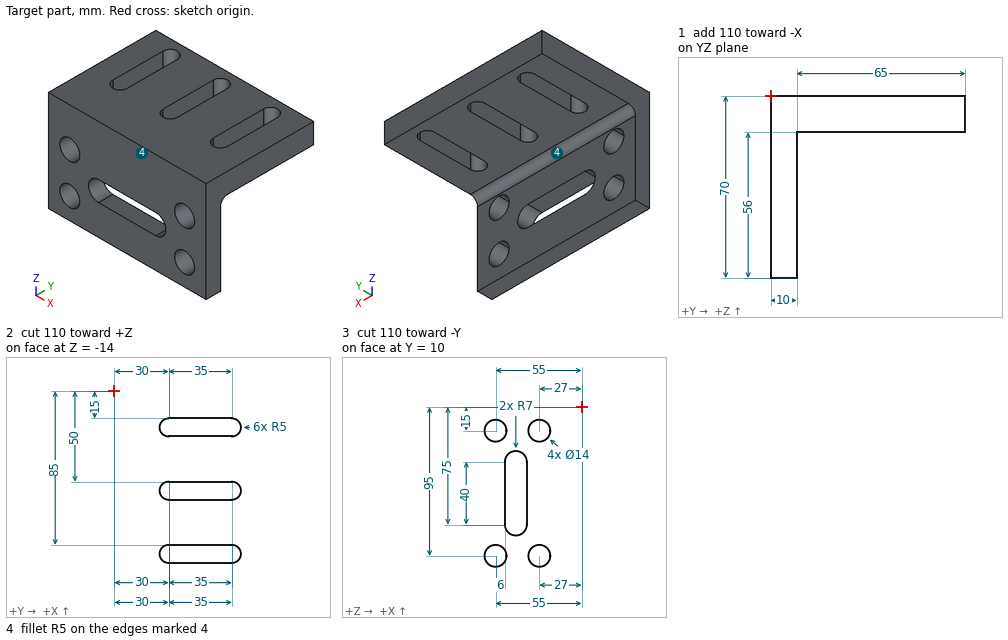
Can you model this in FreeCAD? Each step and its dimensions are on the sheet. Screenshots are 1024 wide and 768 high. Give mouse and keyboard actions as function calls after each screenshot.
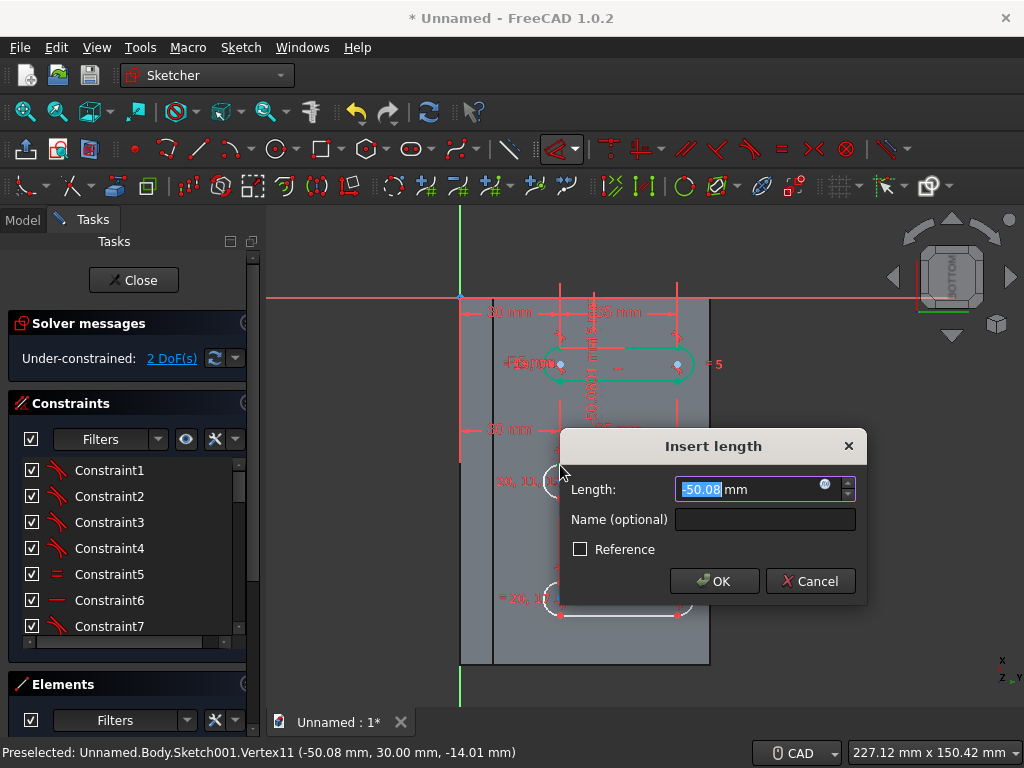
text(-50)
key(Return)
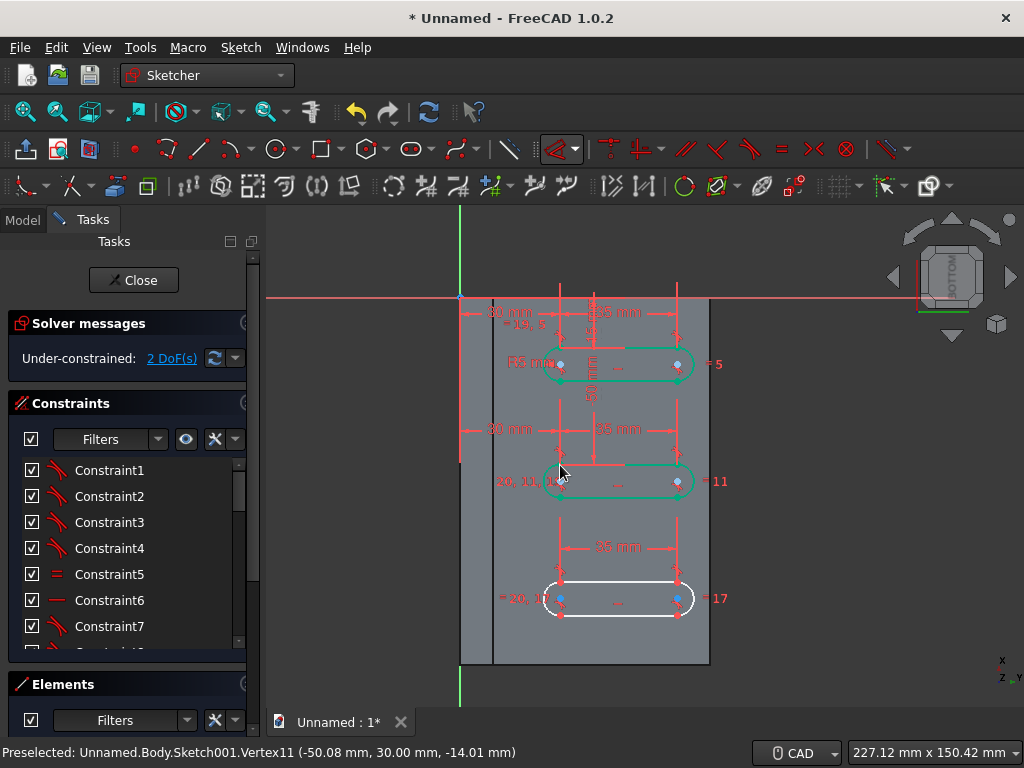
click(560, 582)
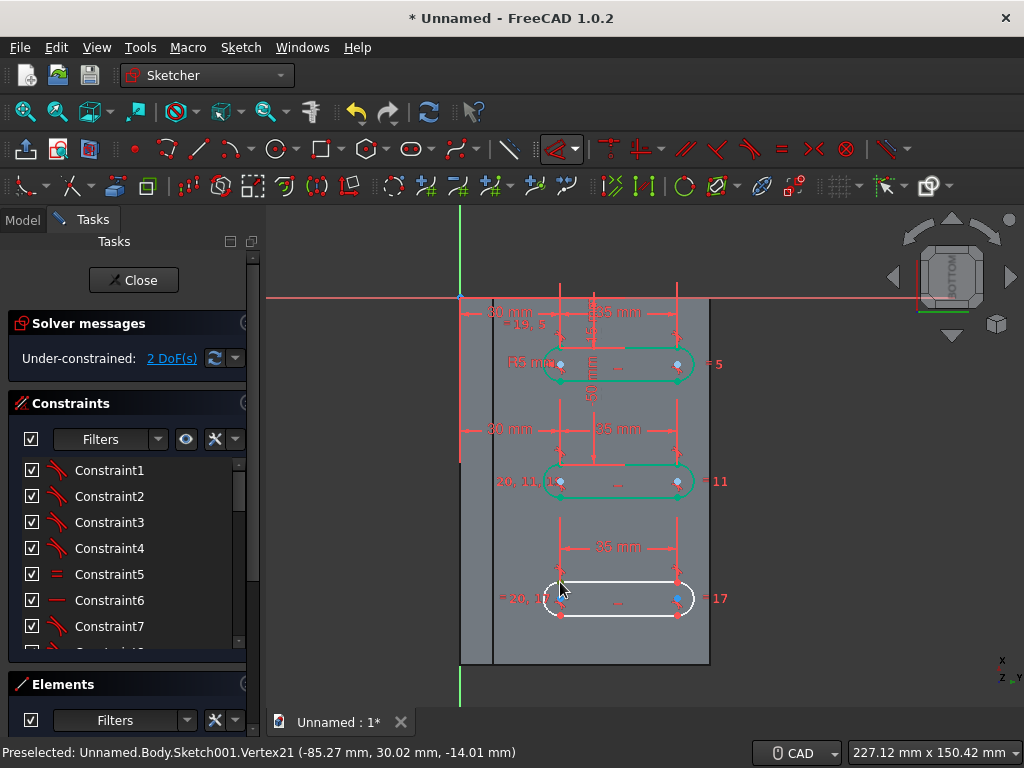
key(l)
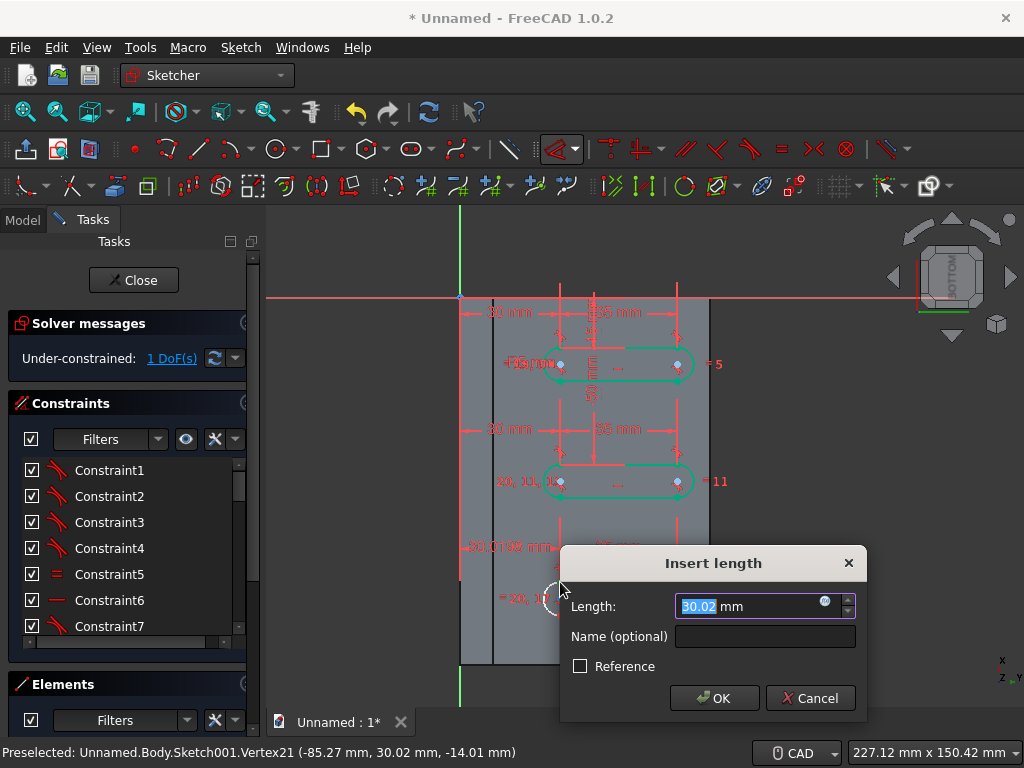
text(30)
key(Return)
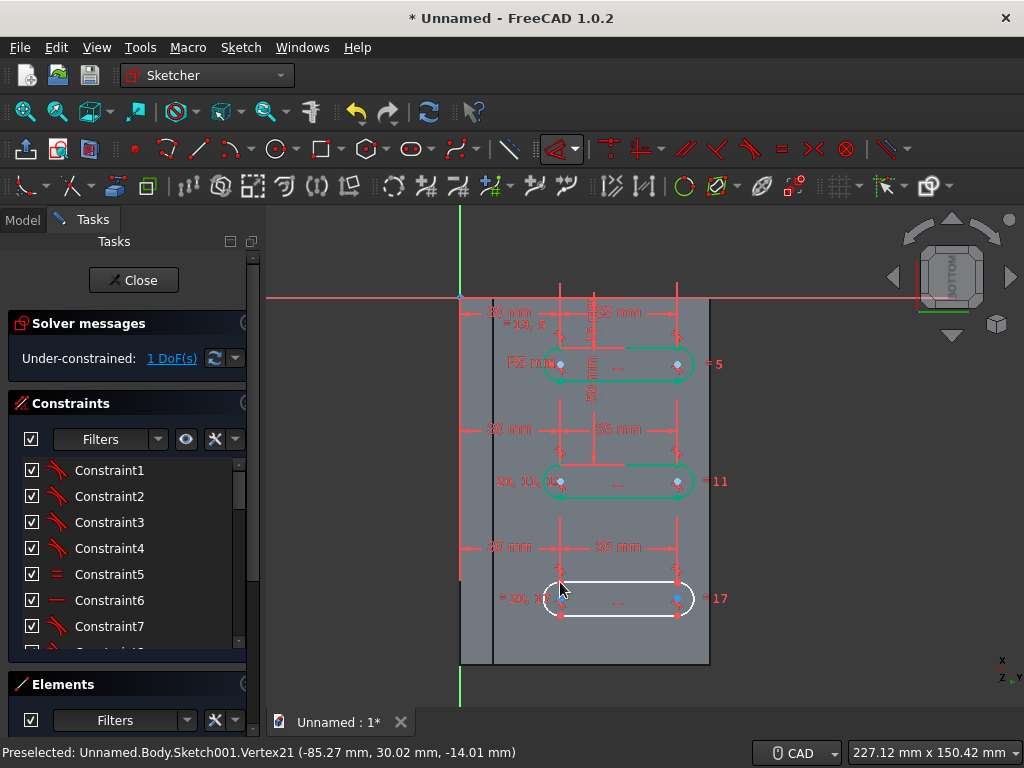
click(560, 582)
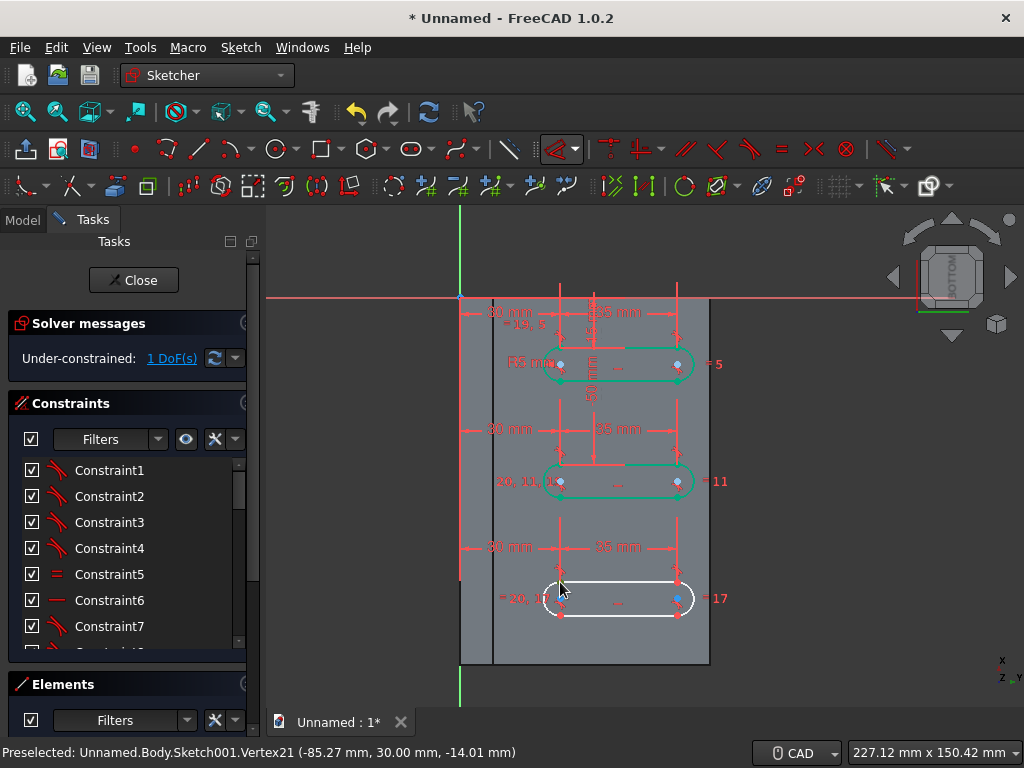
click(578, 150)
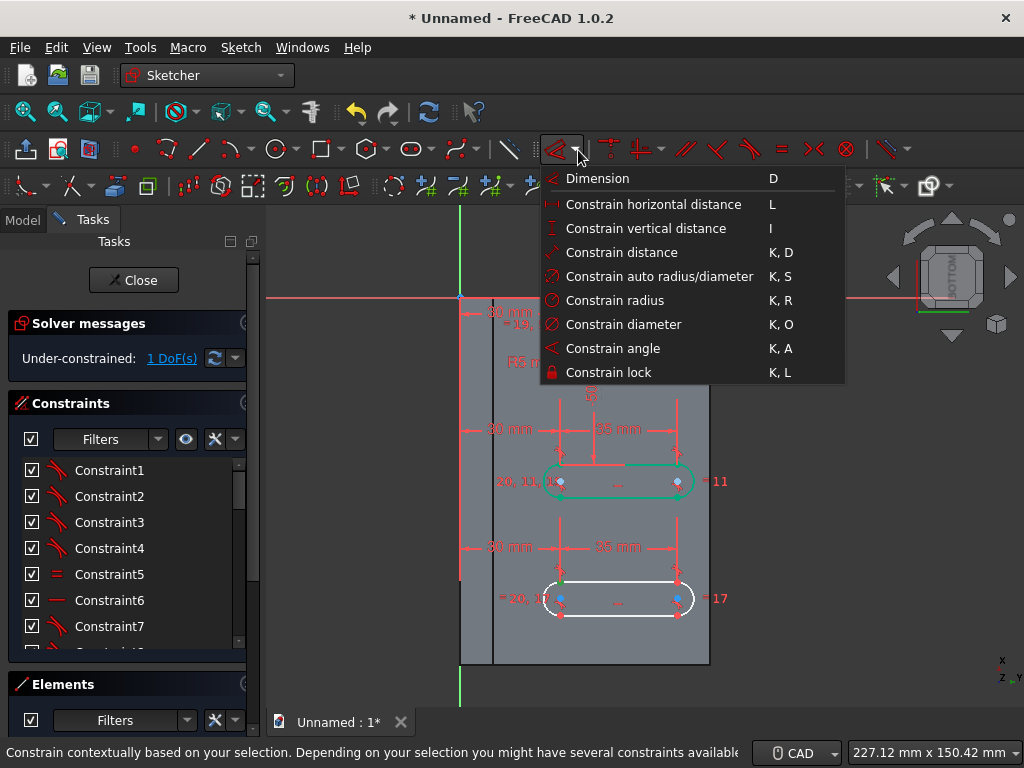
click(693, 228)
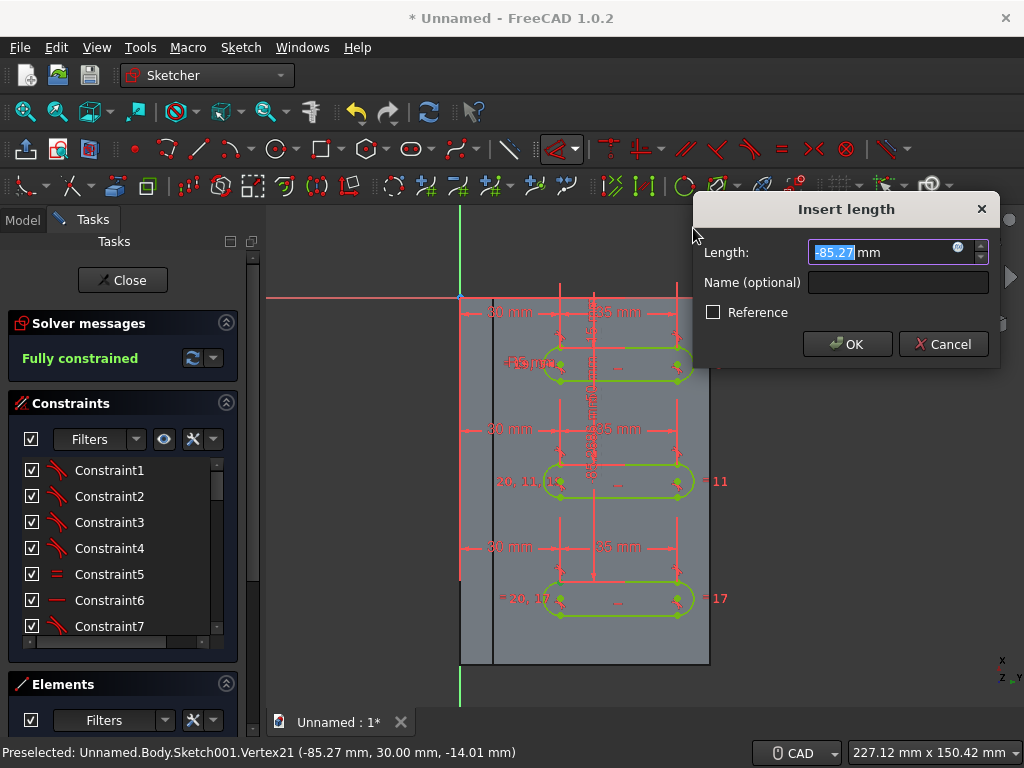
text(-85)
key(Return)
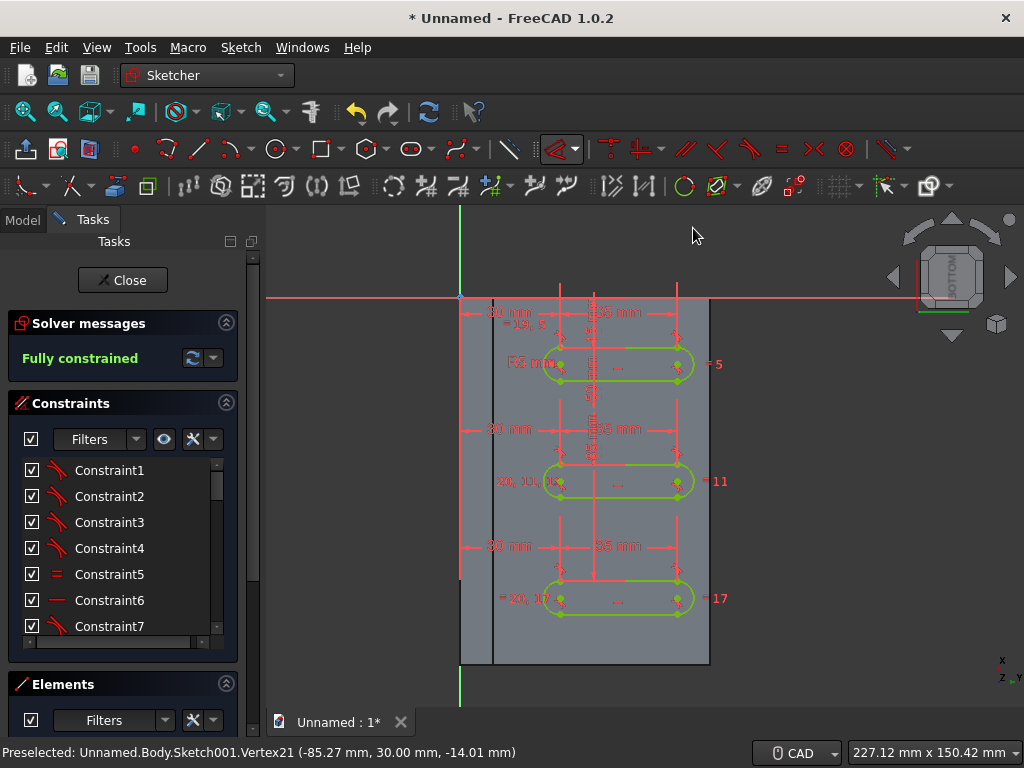
click(123, 280)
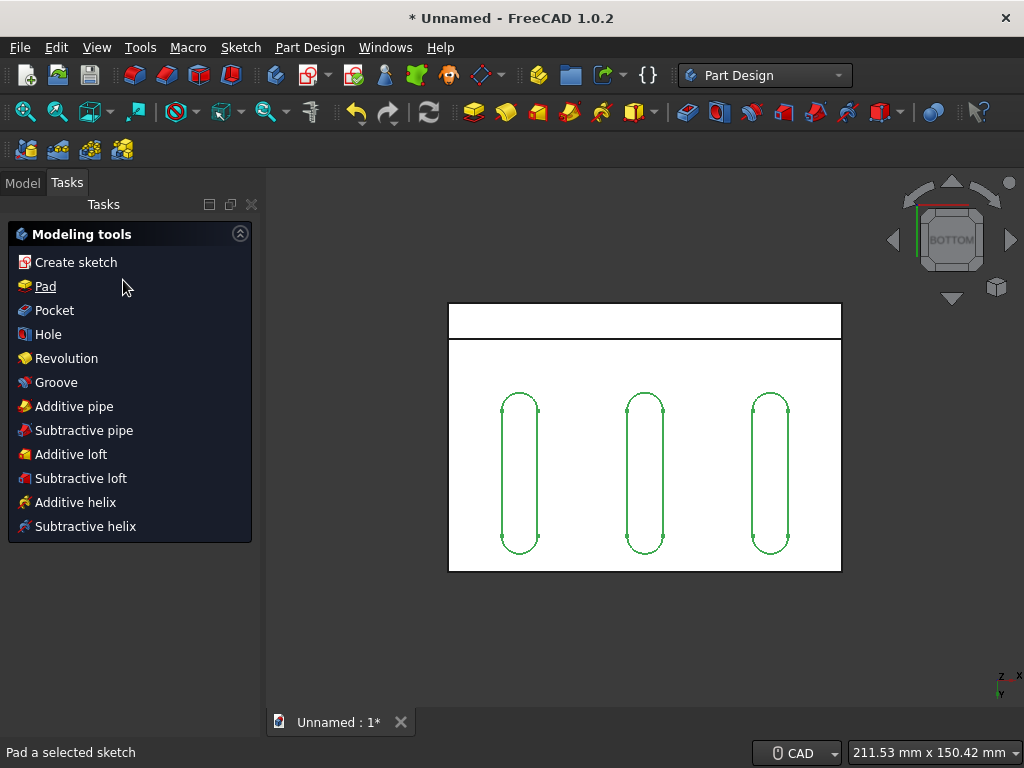
click(688, 112)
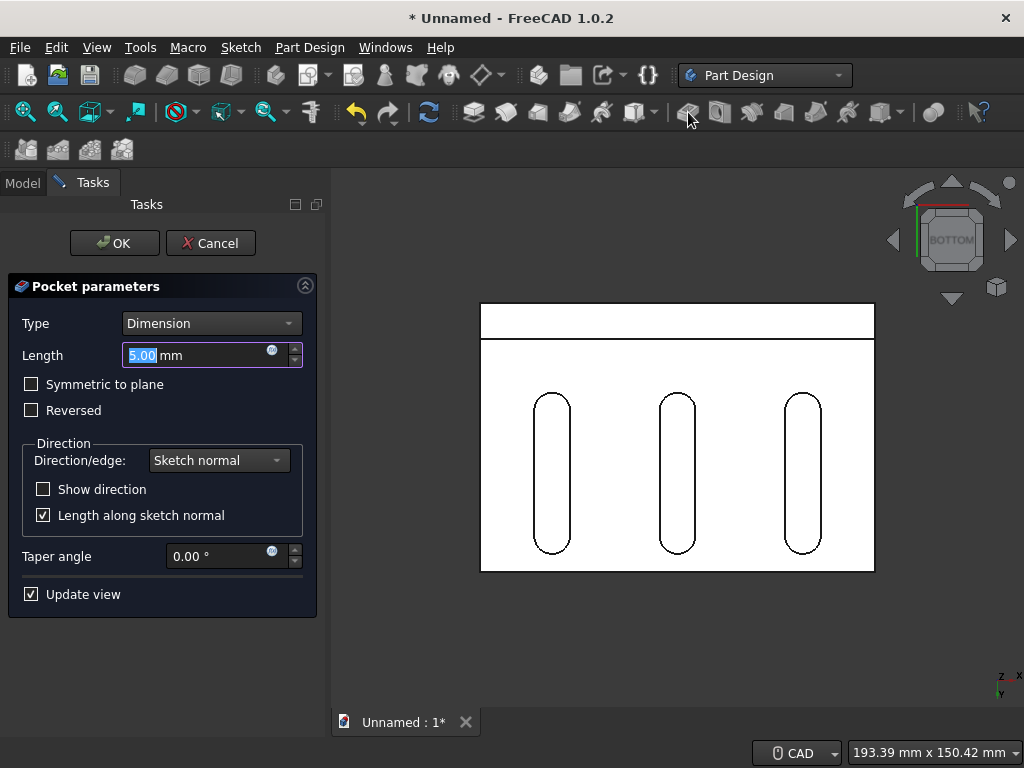
text(110)
key(Tab)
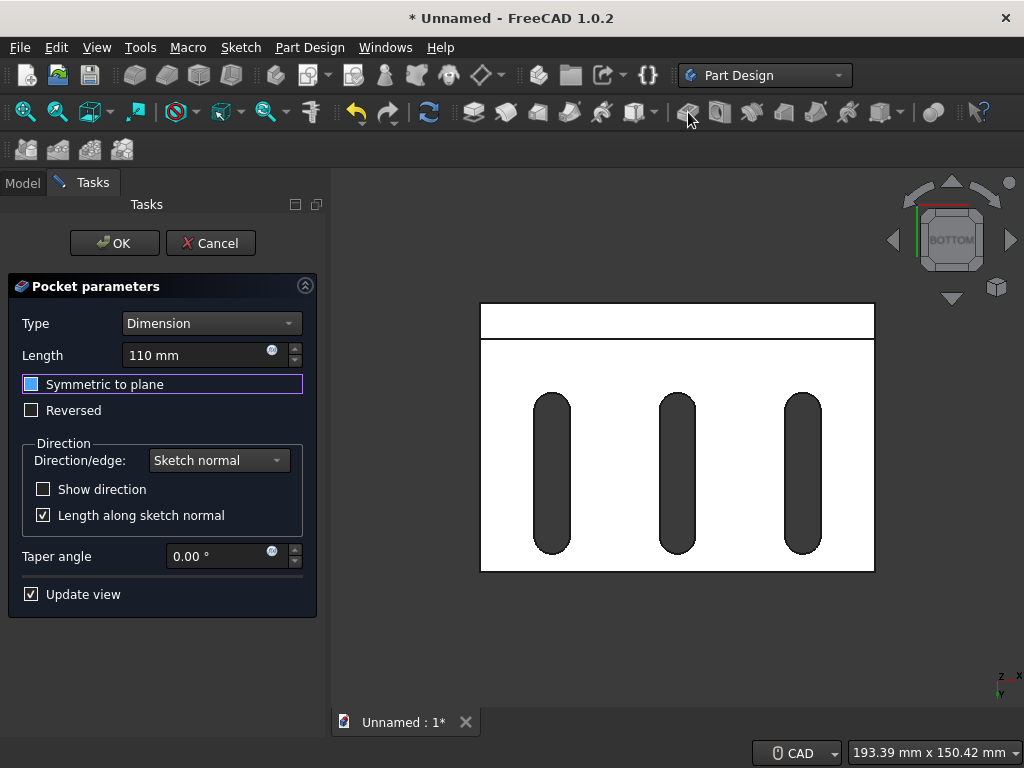
click(115, 243)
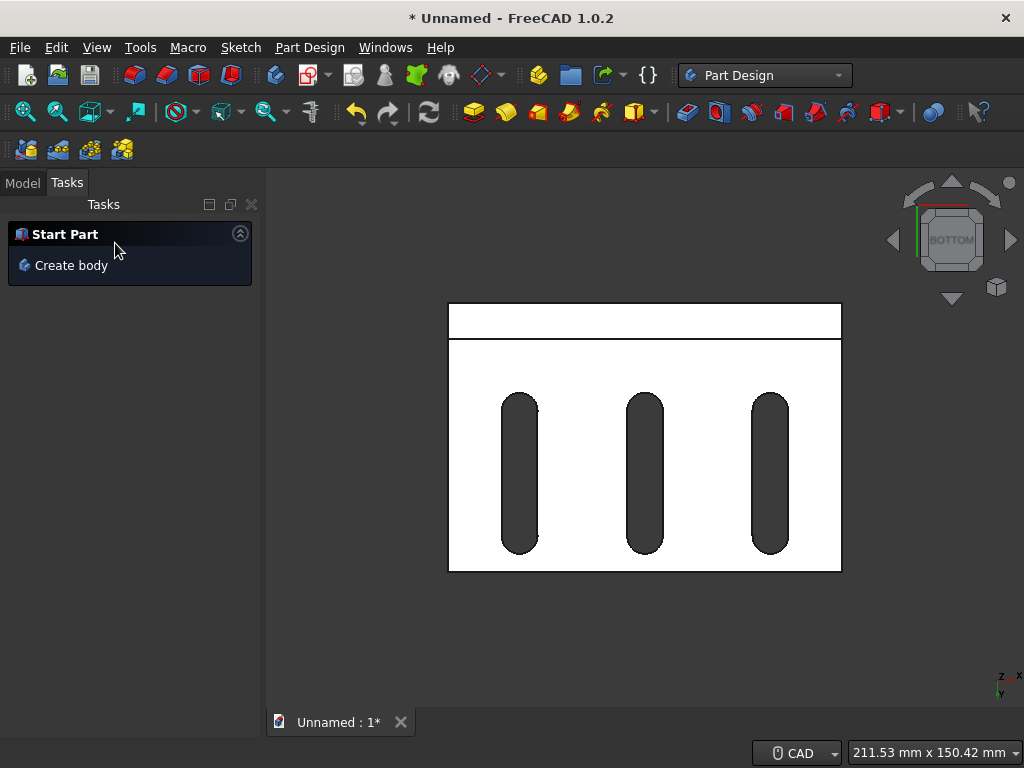
key(4)